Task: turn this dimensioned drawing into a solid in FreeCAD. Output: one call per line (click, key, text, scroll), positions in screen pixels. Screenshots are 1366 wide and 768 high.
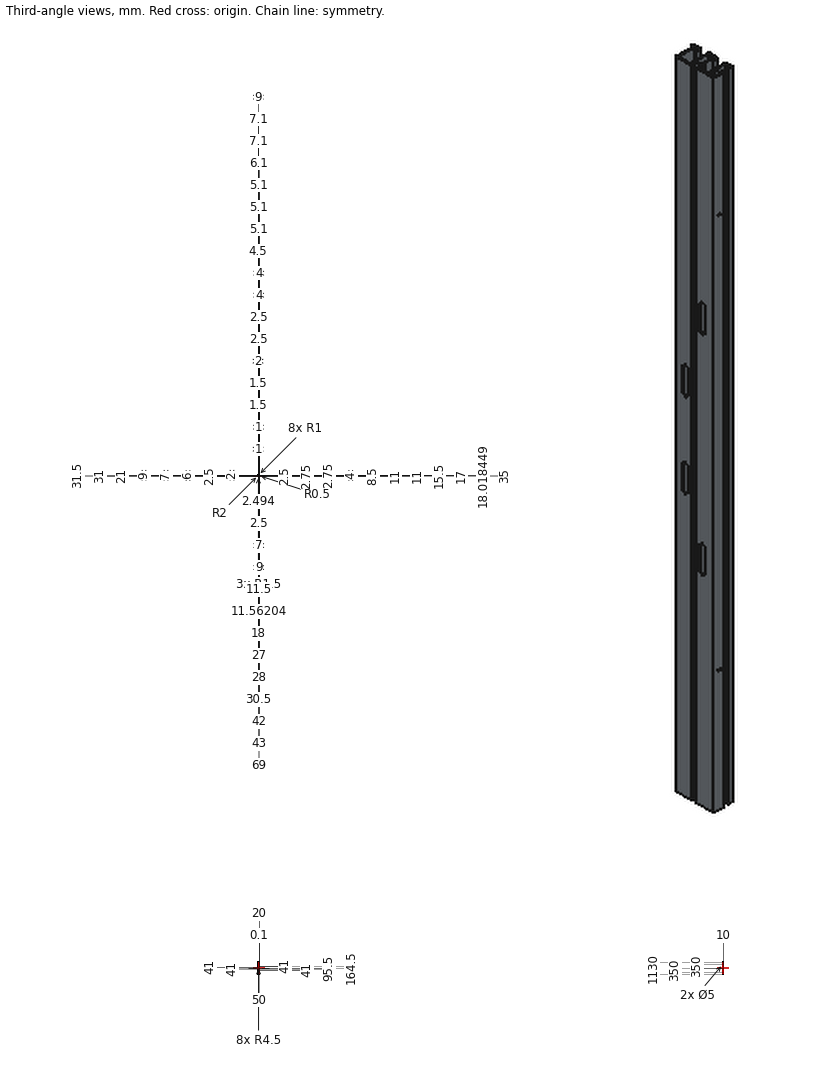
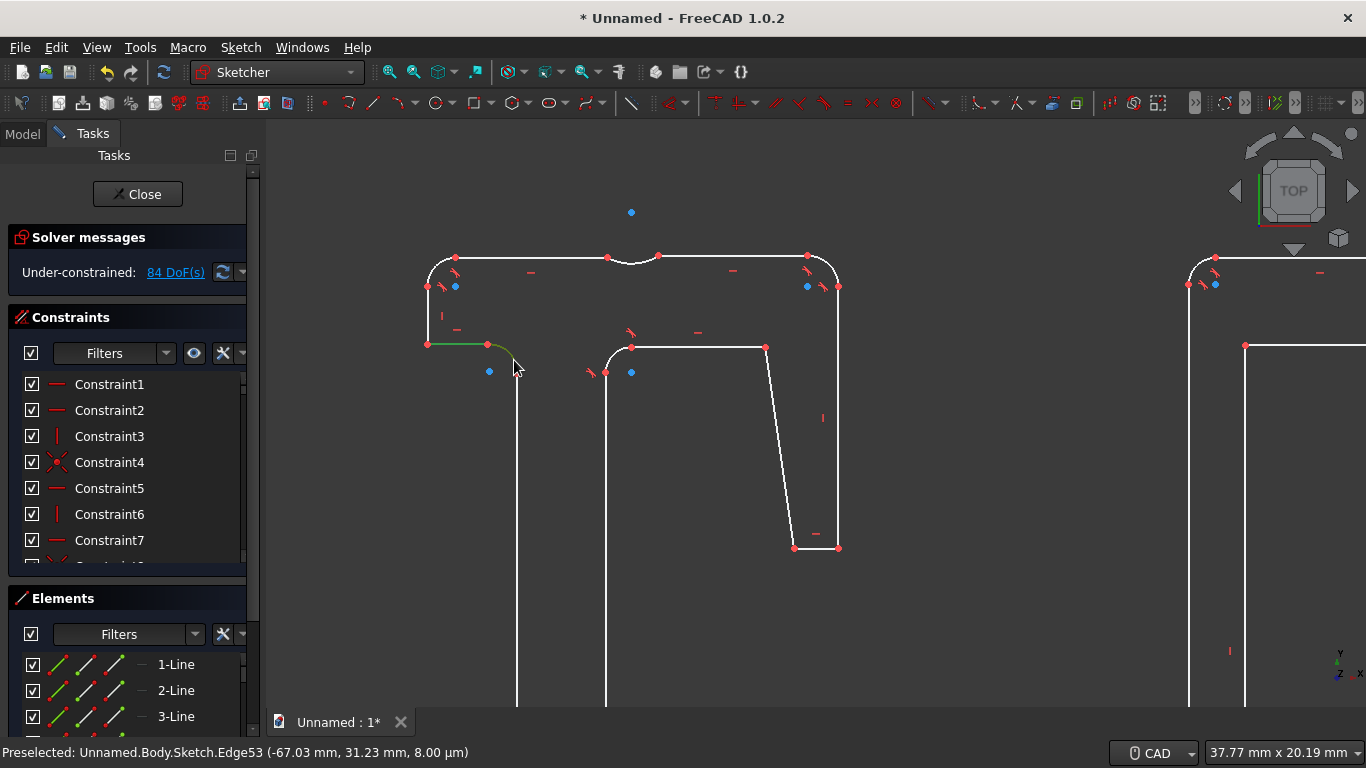
key(t)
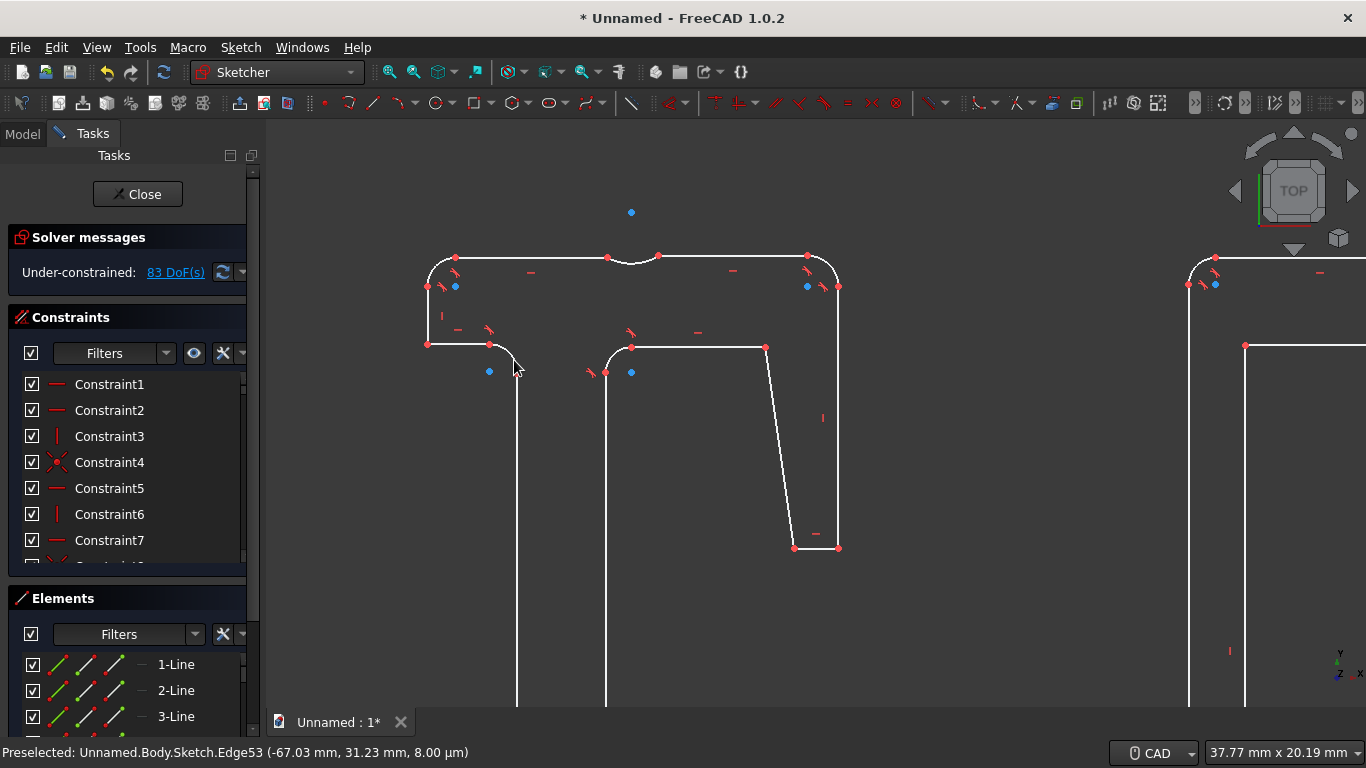
click(517, 644)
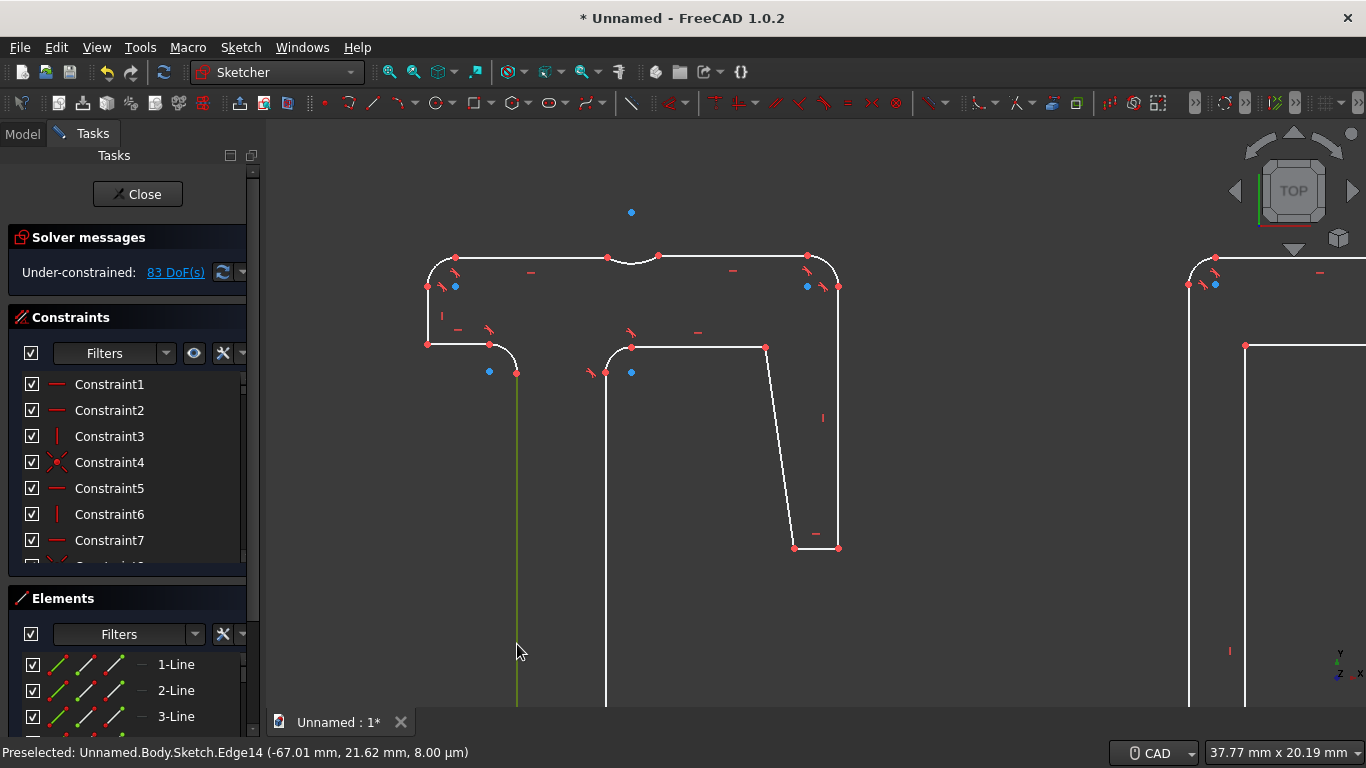
click(514, 360)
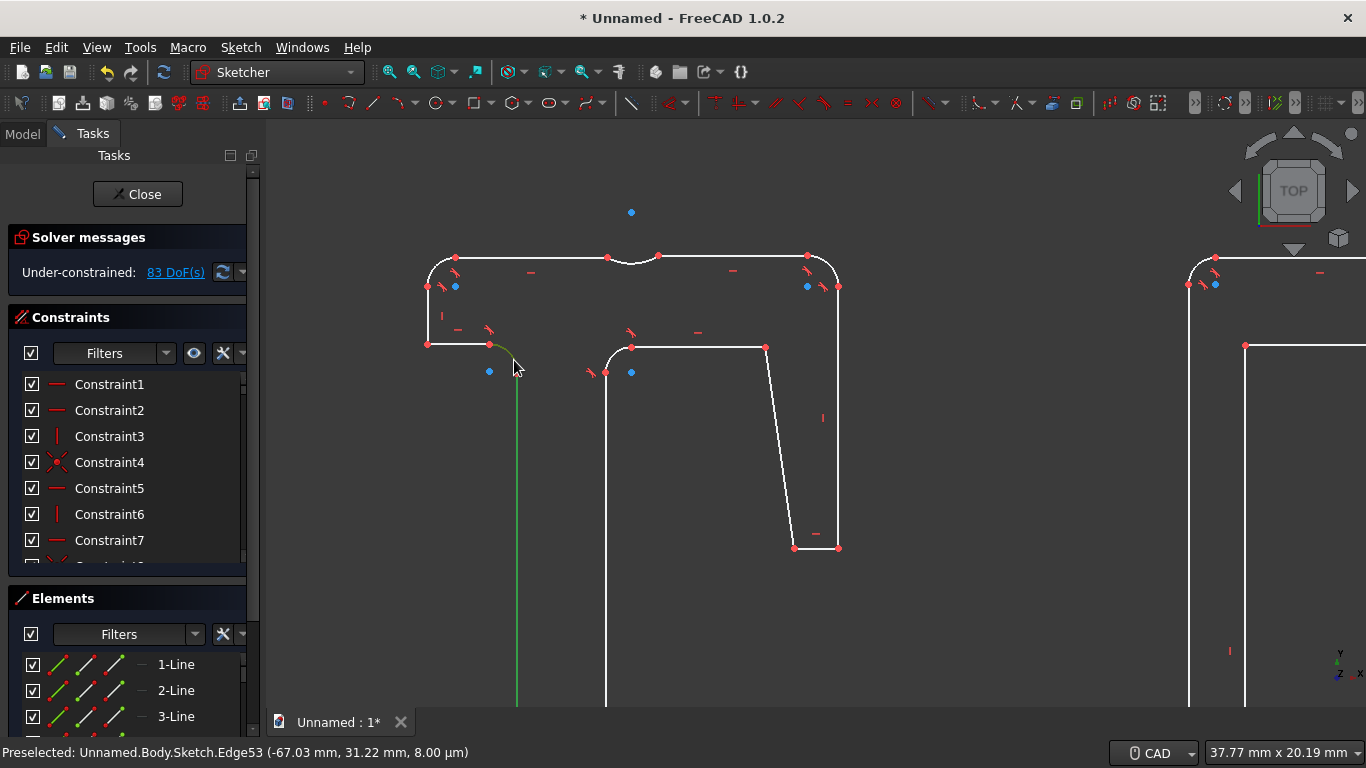
key(t)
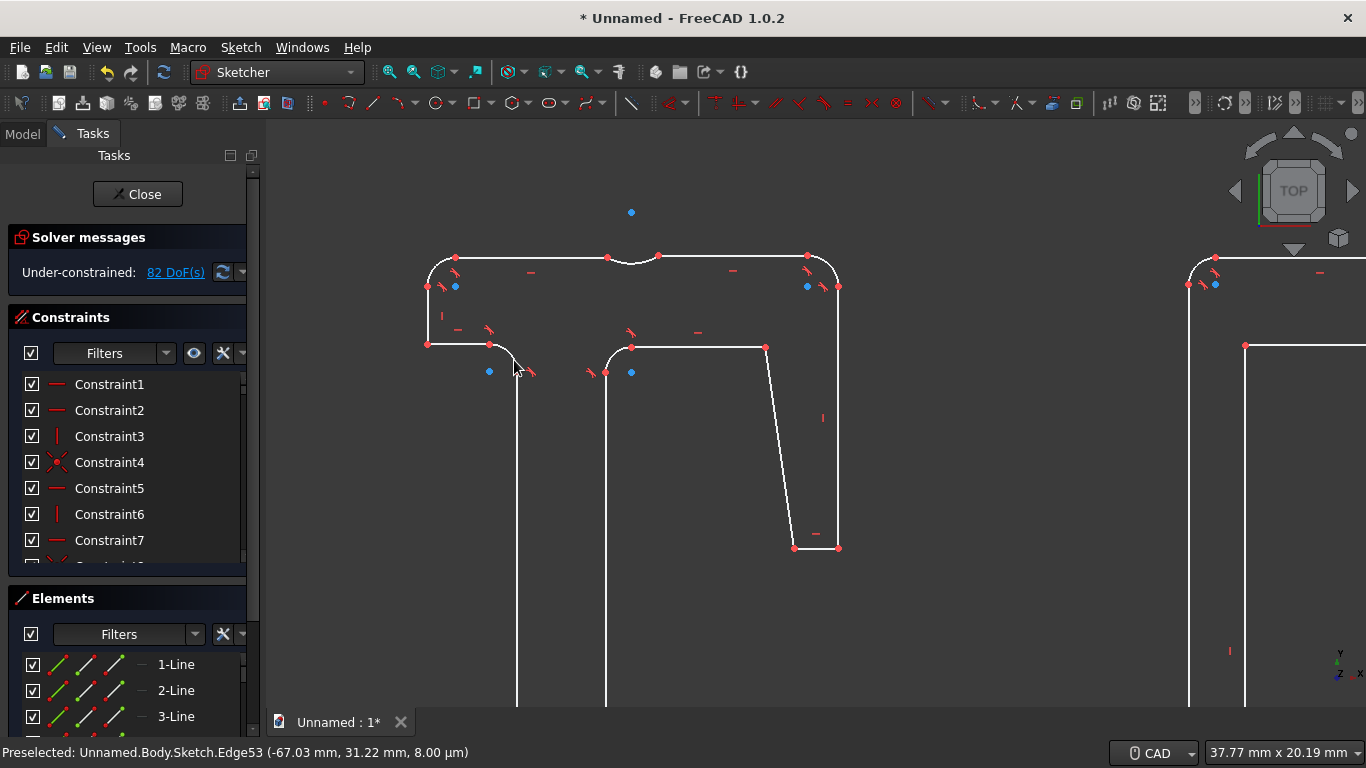
scroll(445, 261, down, 6)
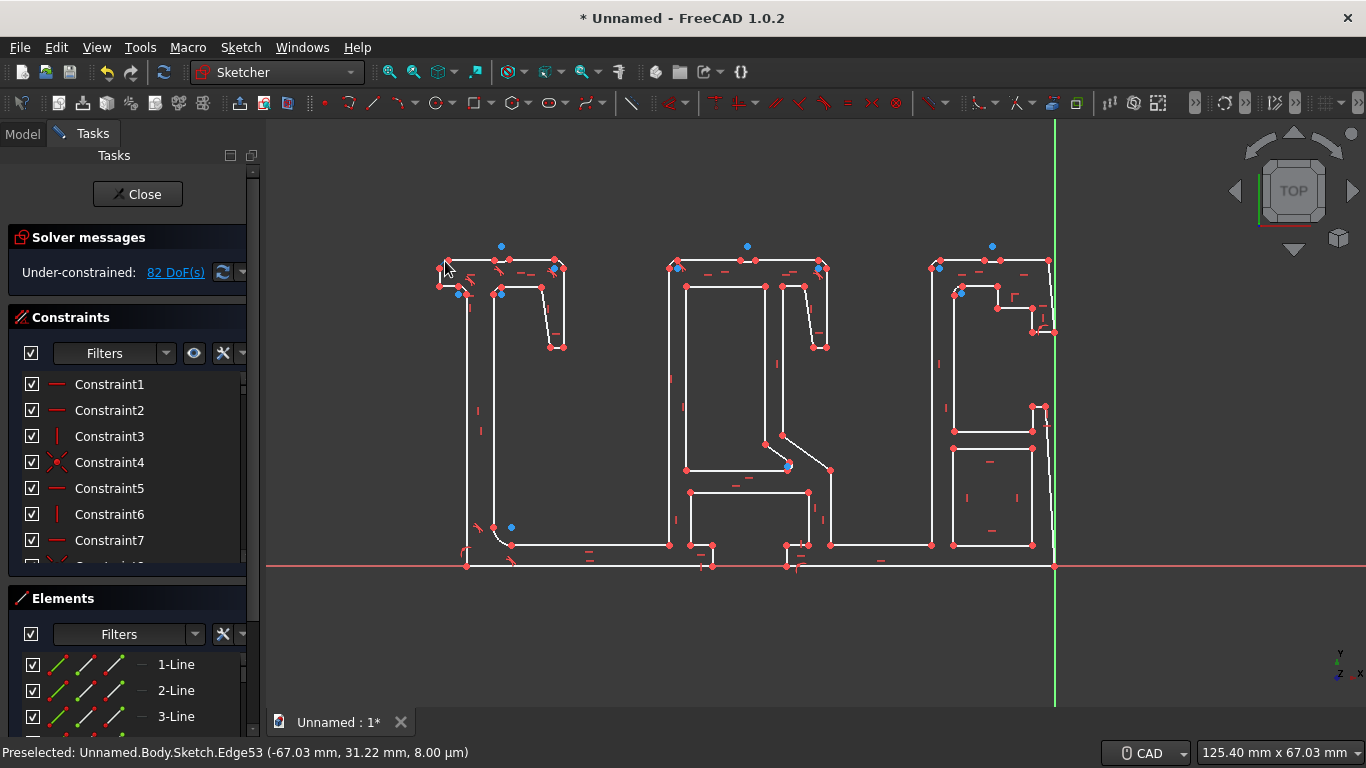
click(954, 391)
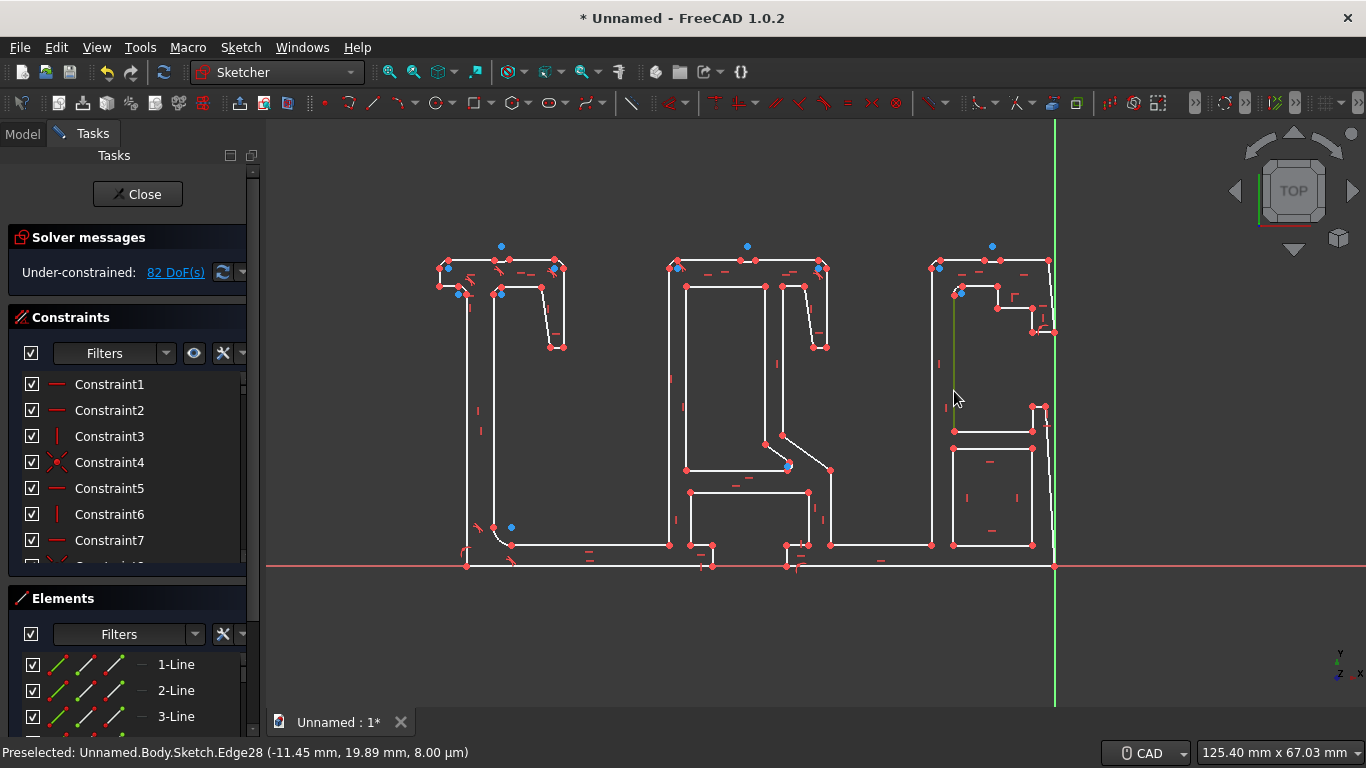
scroll(956, 289, up, 4)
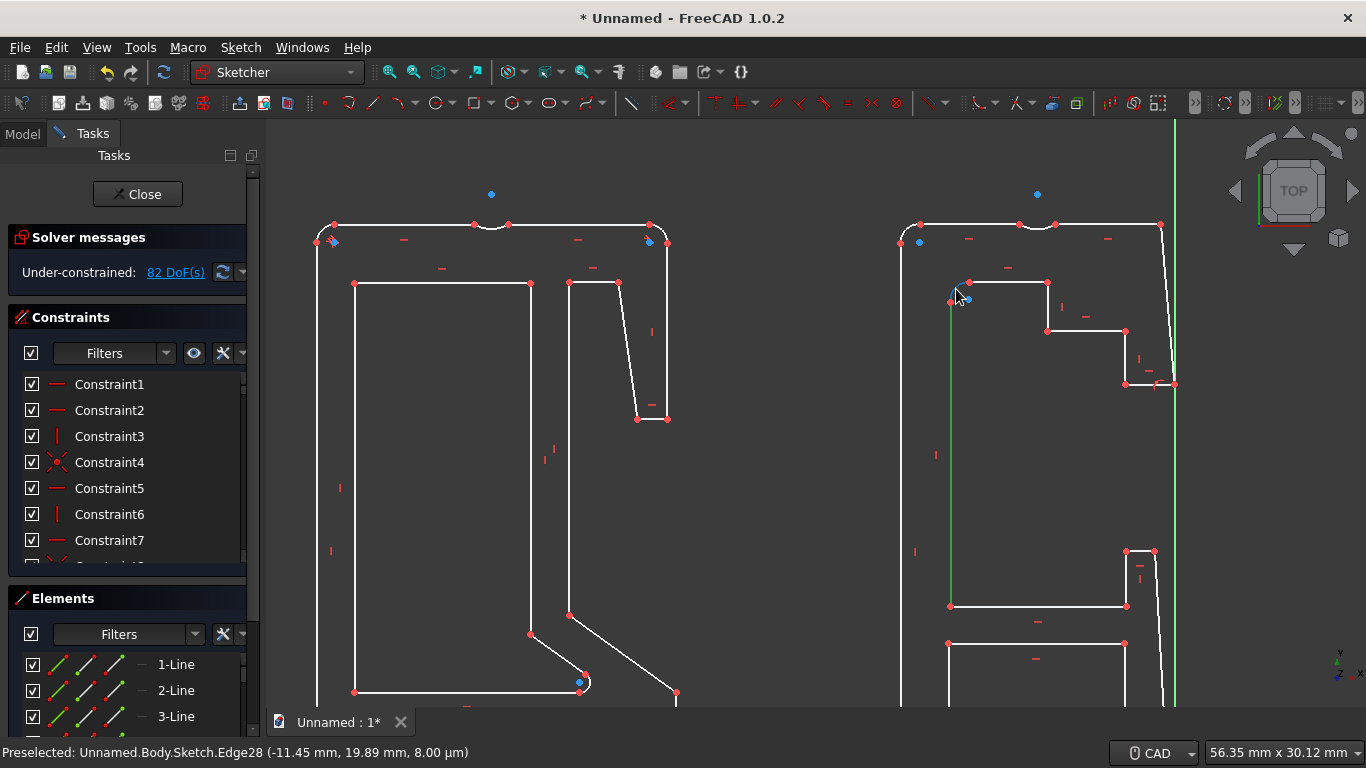
click(955, 288)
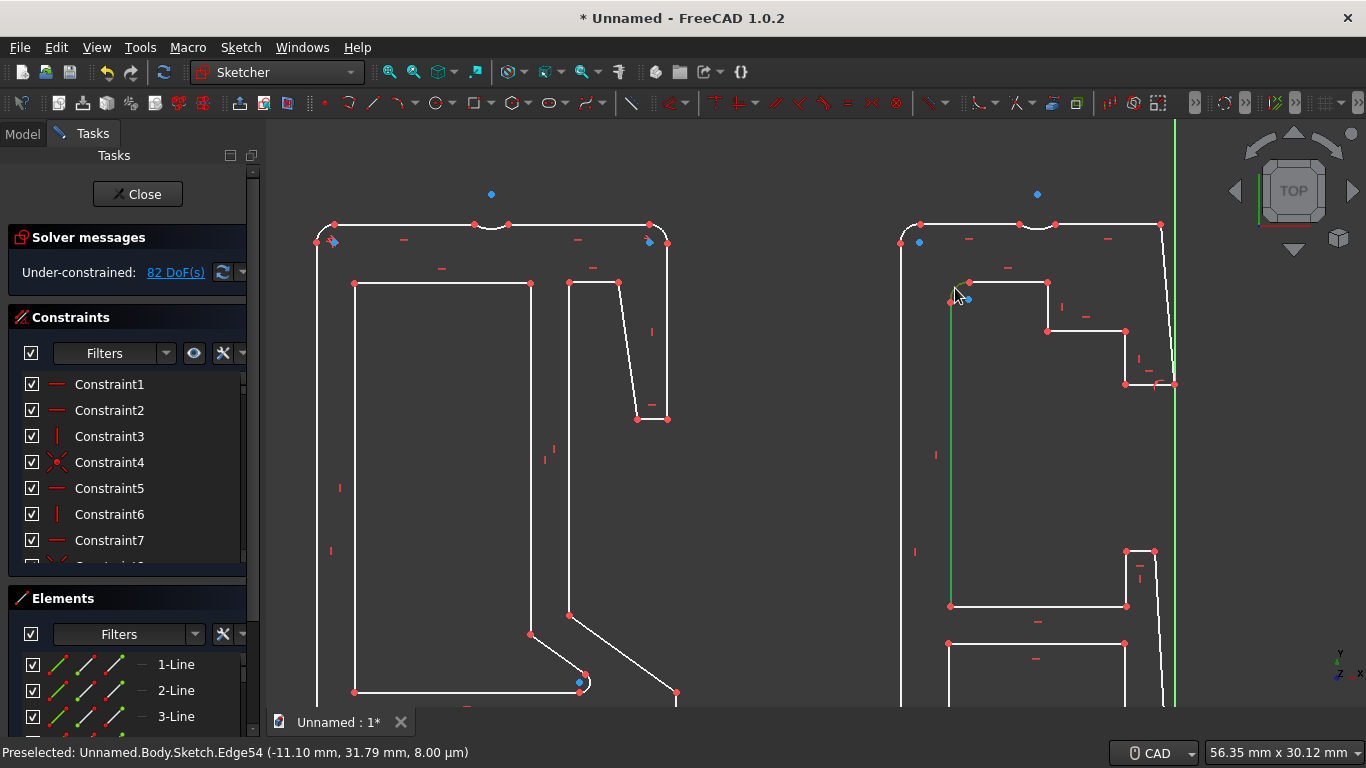
click(824, 104)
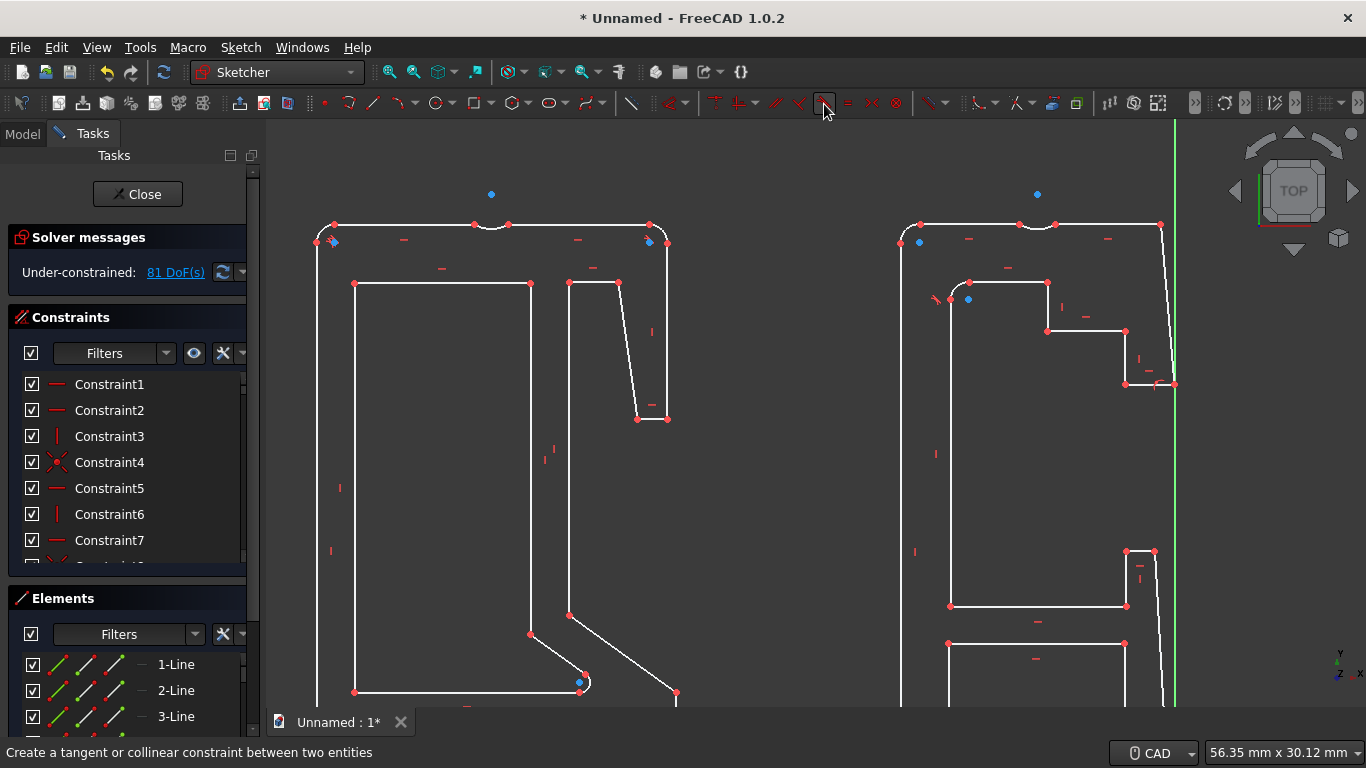
click(993, 282)